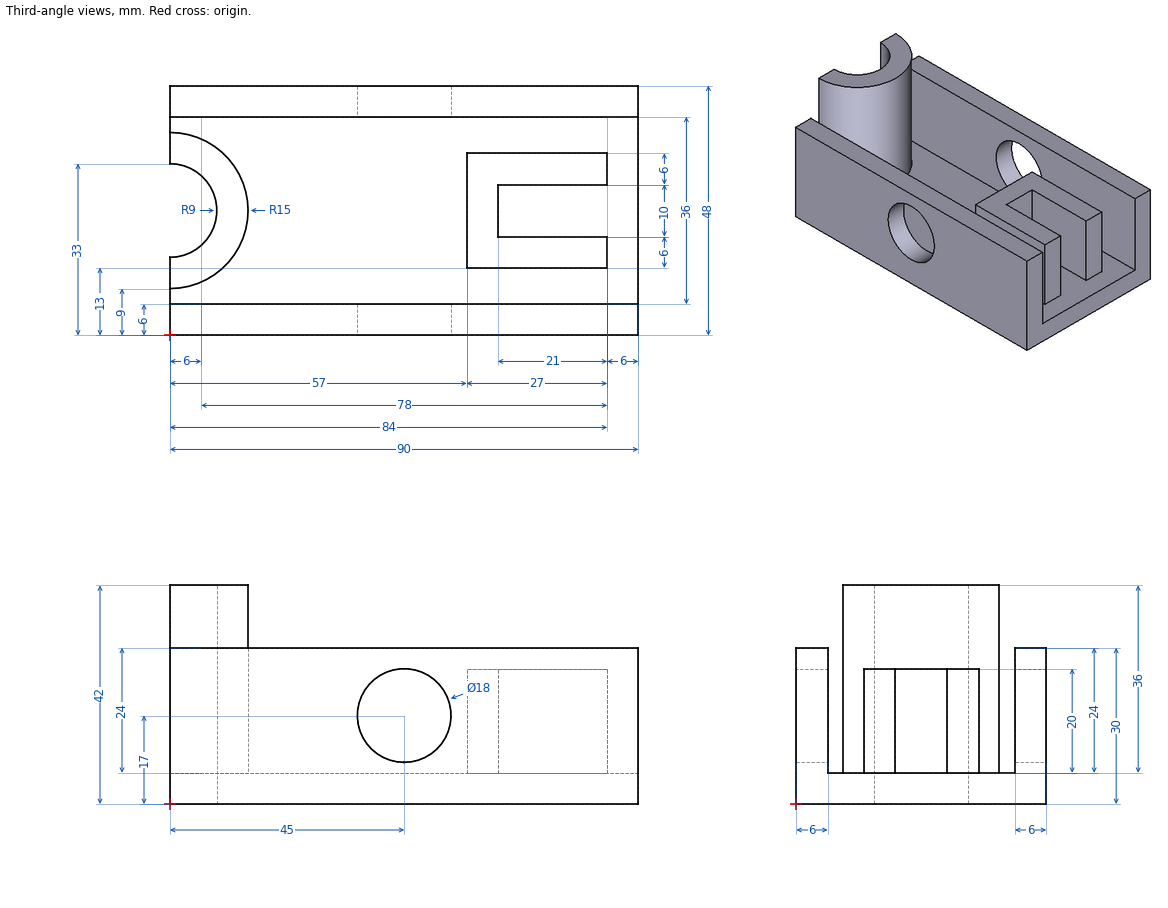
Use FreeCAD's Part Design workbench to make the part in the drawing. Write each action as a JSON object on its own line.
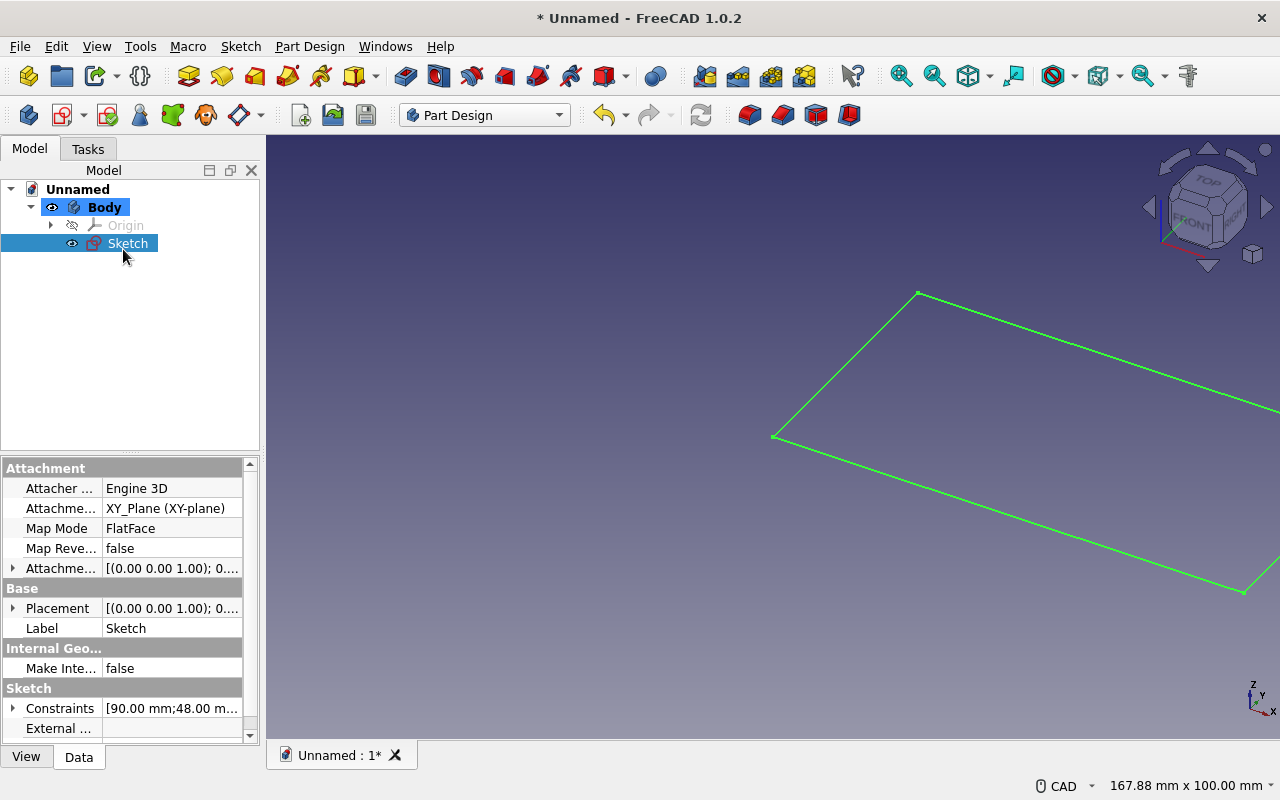
{"action": "left_click", "coordinate": [189, 76]}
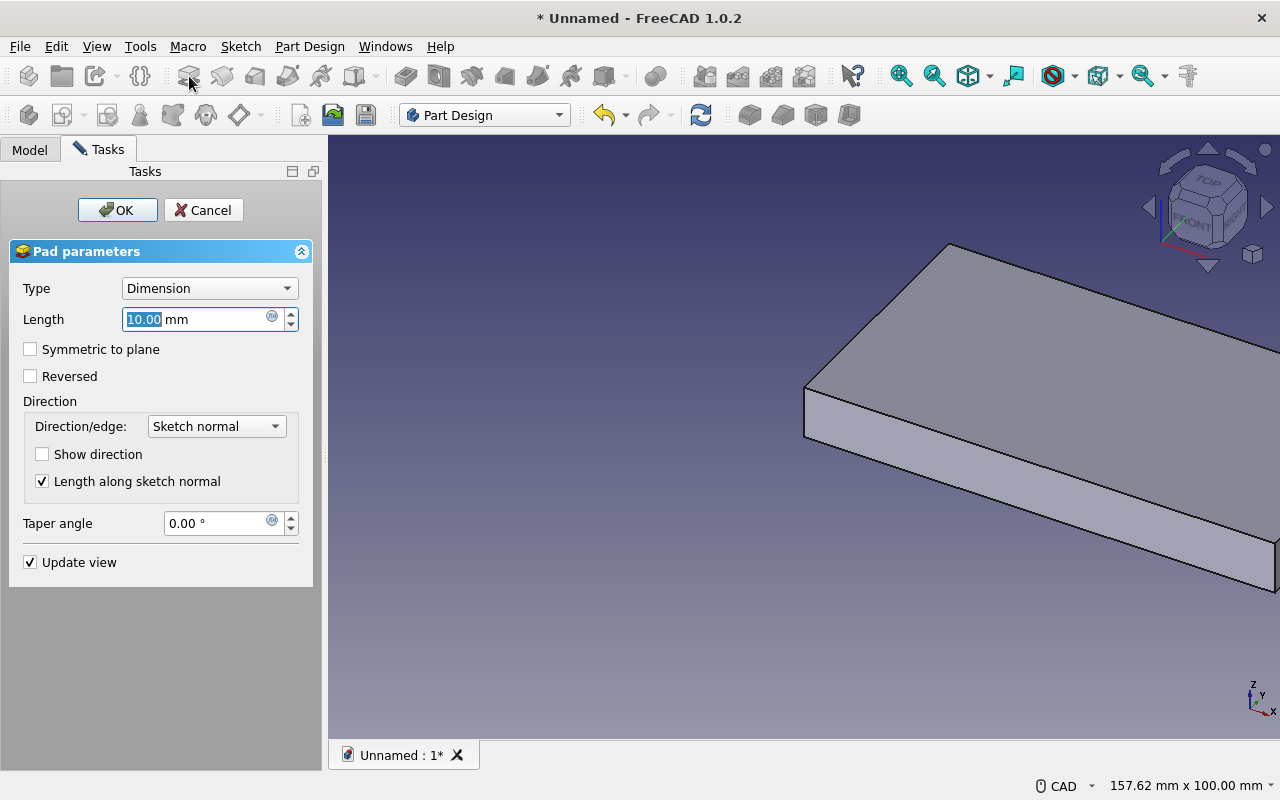
{"action": "type", "text": "30"}
{"action": "key", "text": "Tab"}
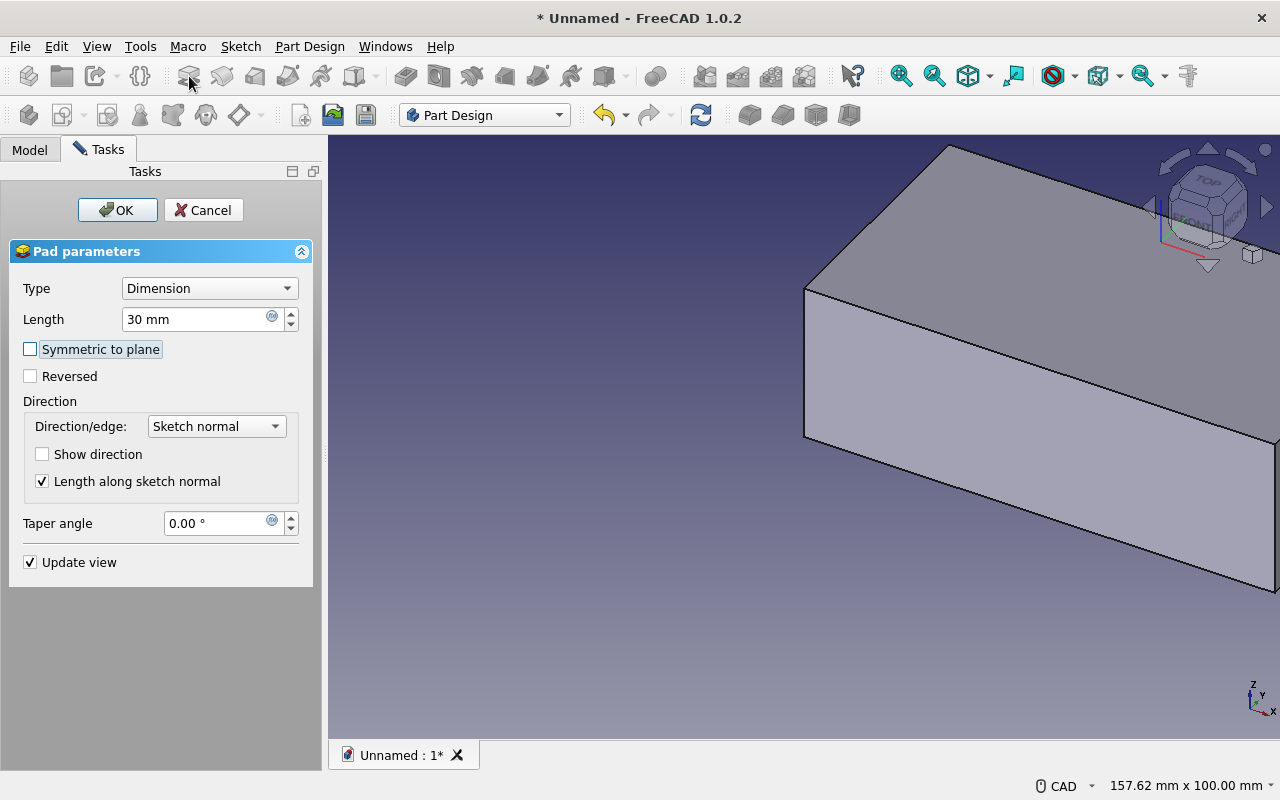
{"action": "left_click", "coordinate": [118, 210]}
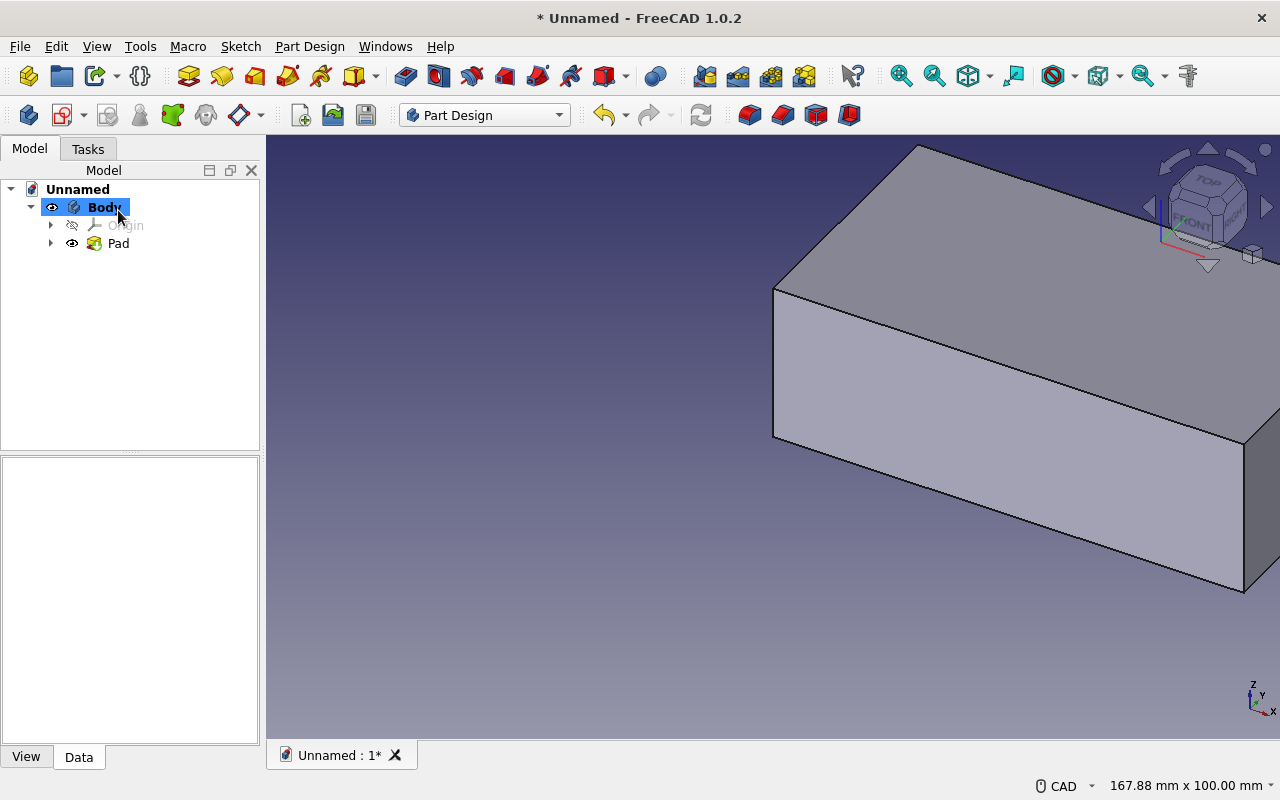
{"action": "left_click", "coordinate": [902, 76]}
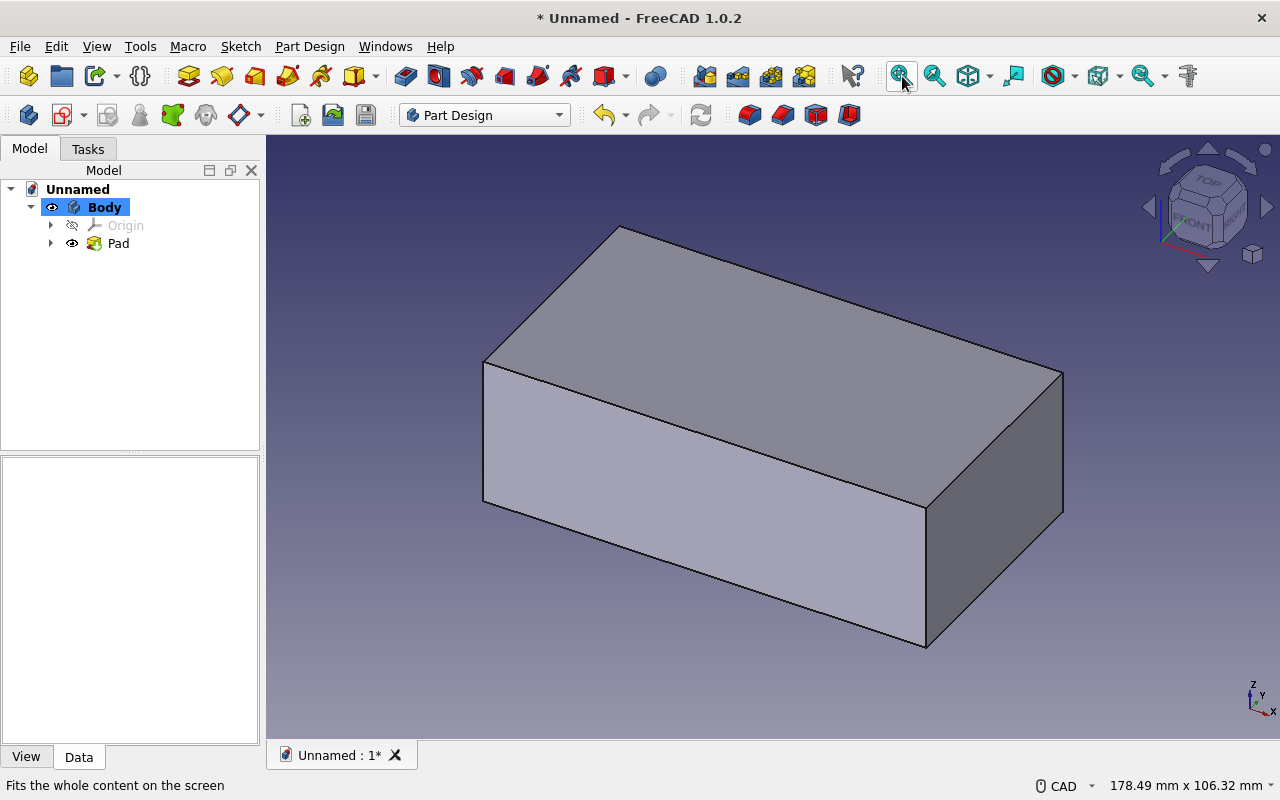
{"action": "left_click", "coordinate": [836, 387]}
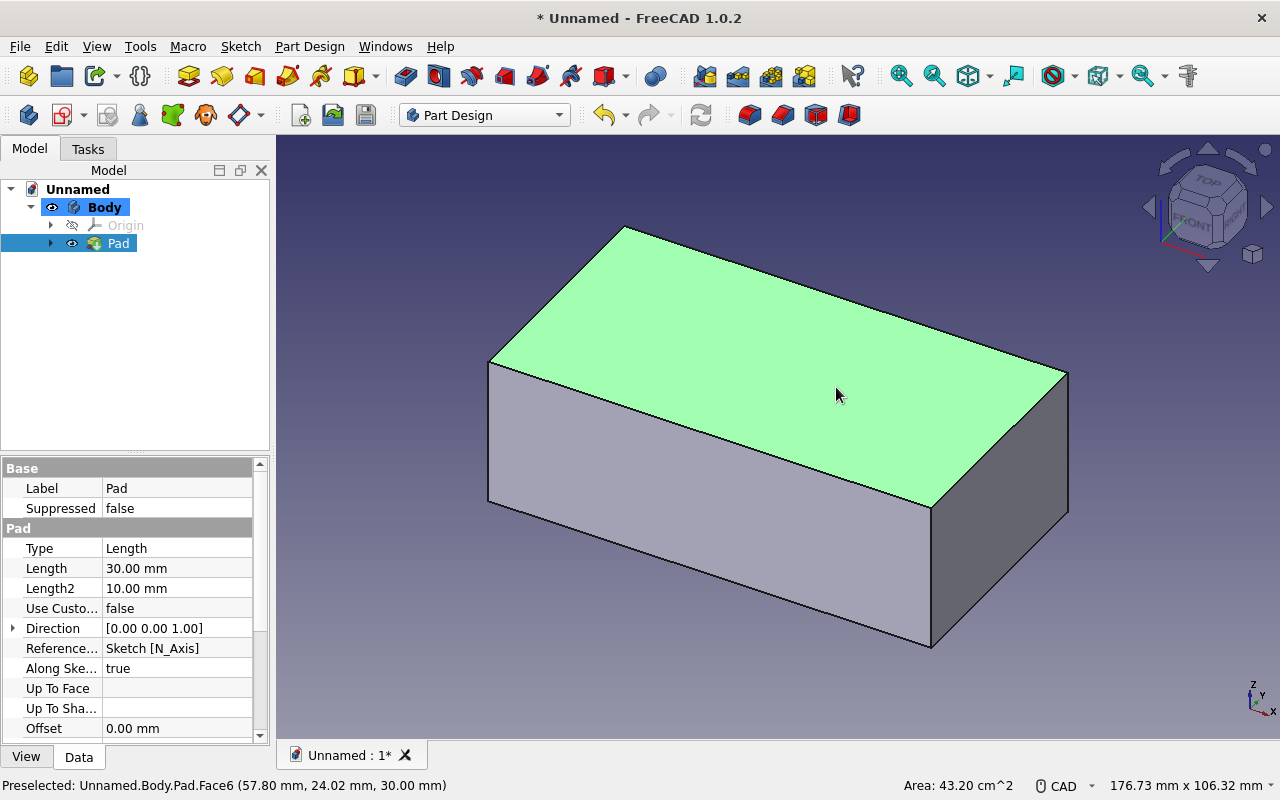
{"action": "left_click", "coordinate": [62, 116]}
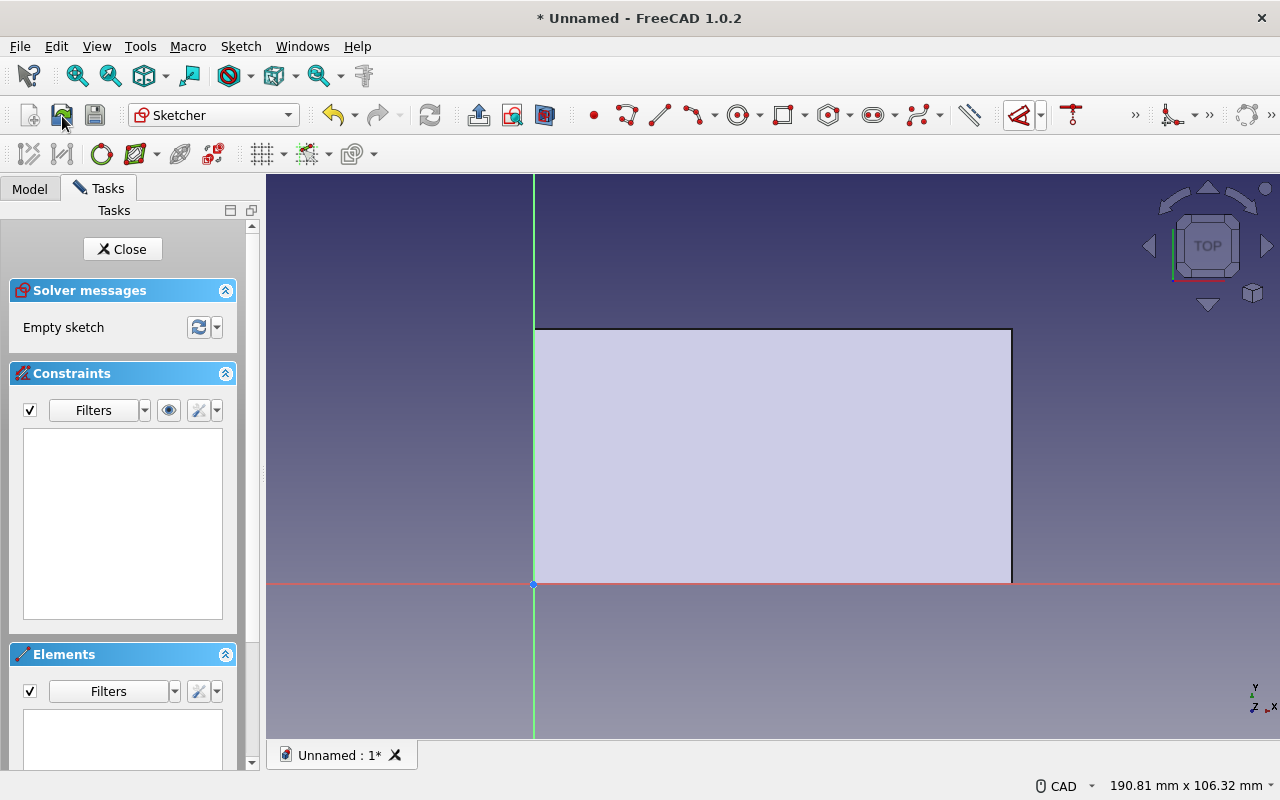
{"action": "key", "text": "g r"}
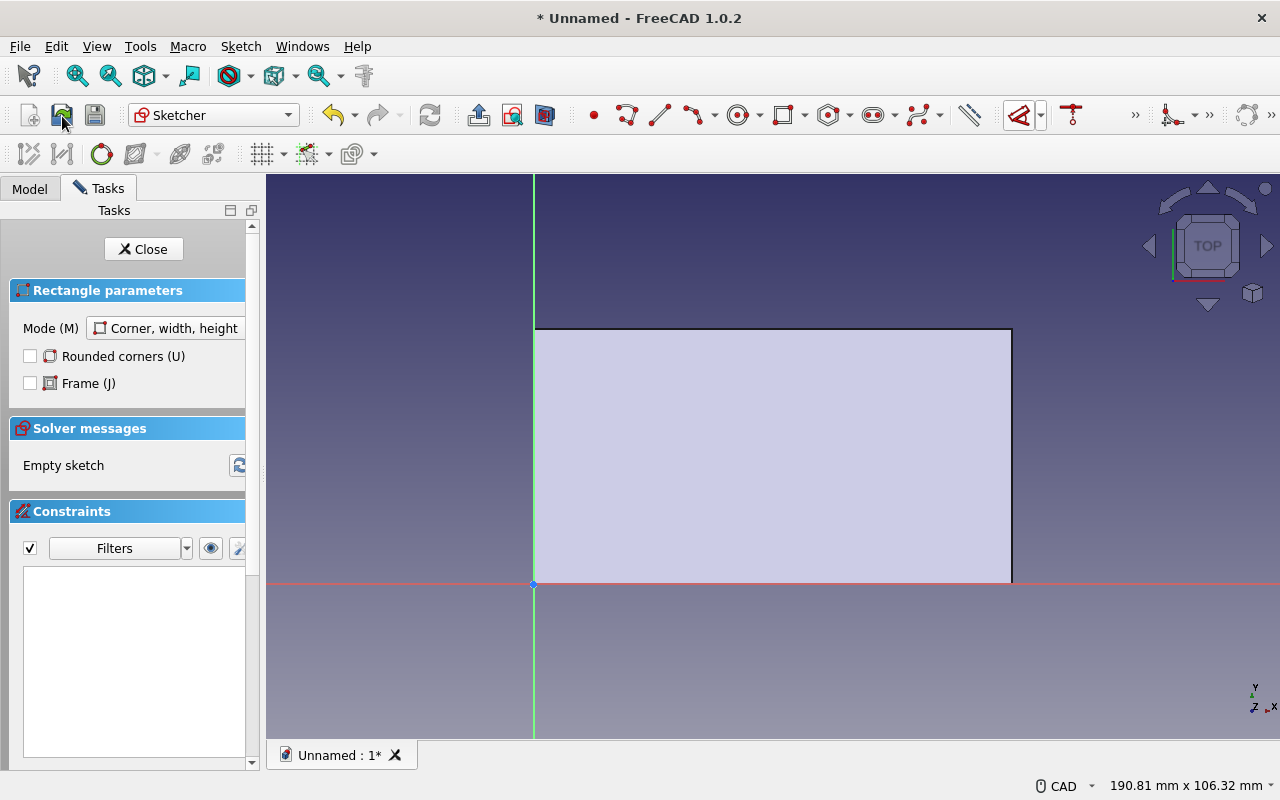
{"action": "left_click", "coordinate": [566, 361]}
{"action": "mouse_move", "coordinate": [980, 552]}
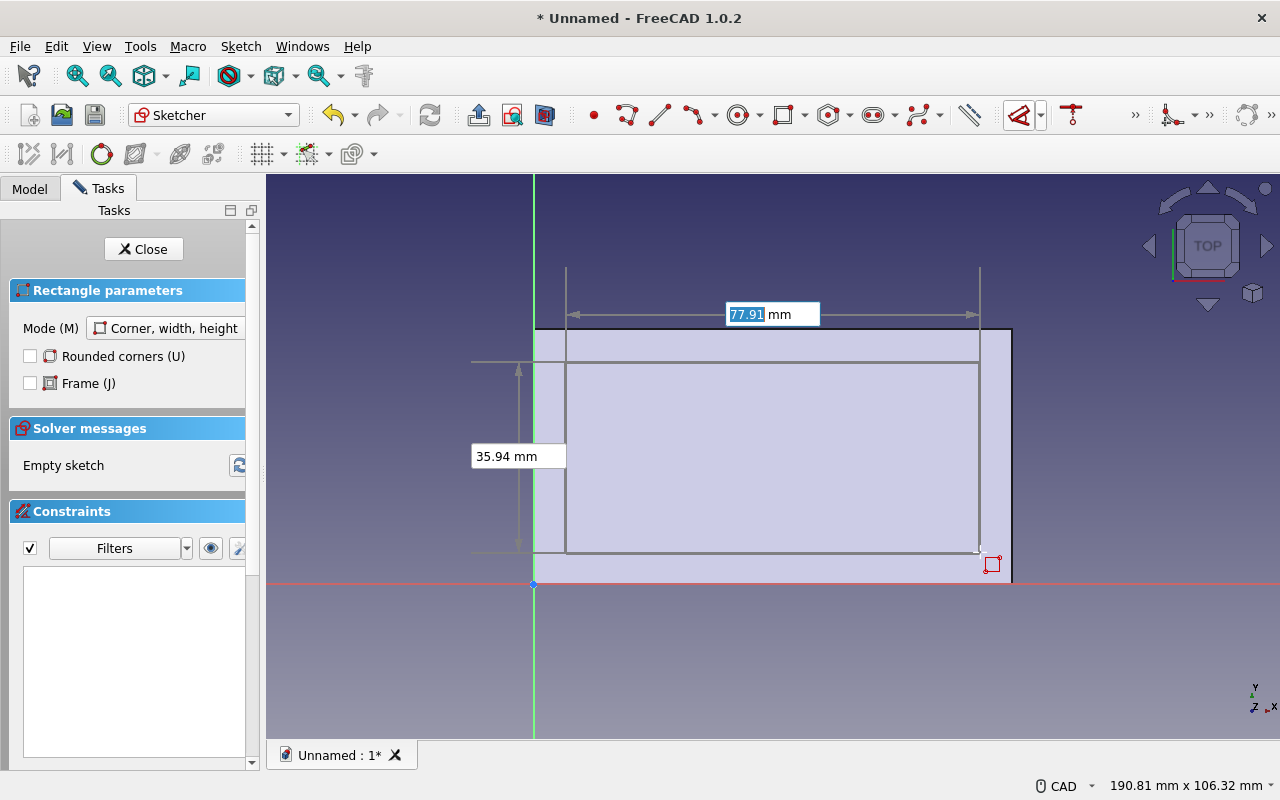
{"action": "type", "text": "78"}
{"action": "key", "text": "Tab"}
{"action": "type", "text": "36"}
{"action": "key", "text": "Return"}
{"action": "key", "text": "Escape"}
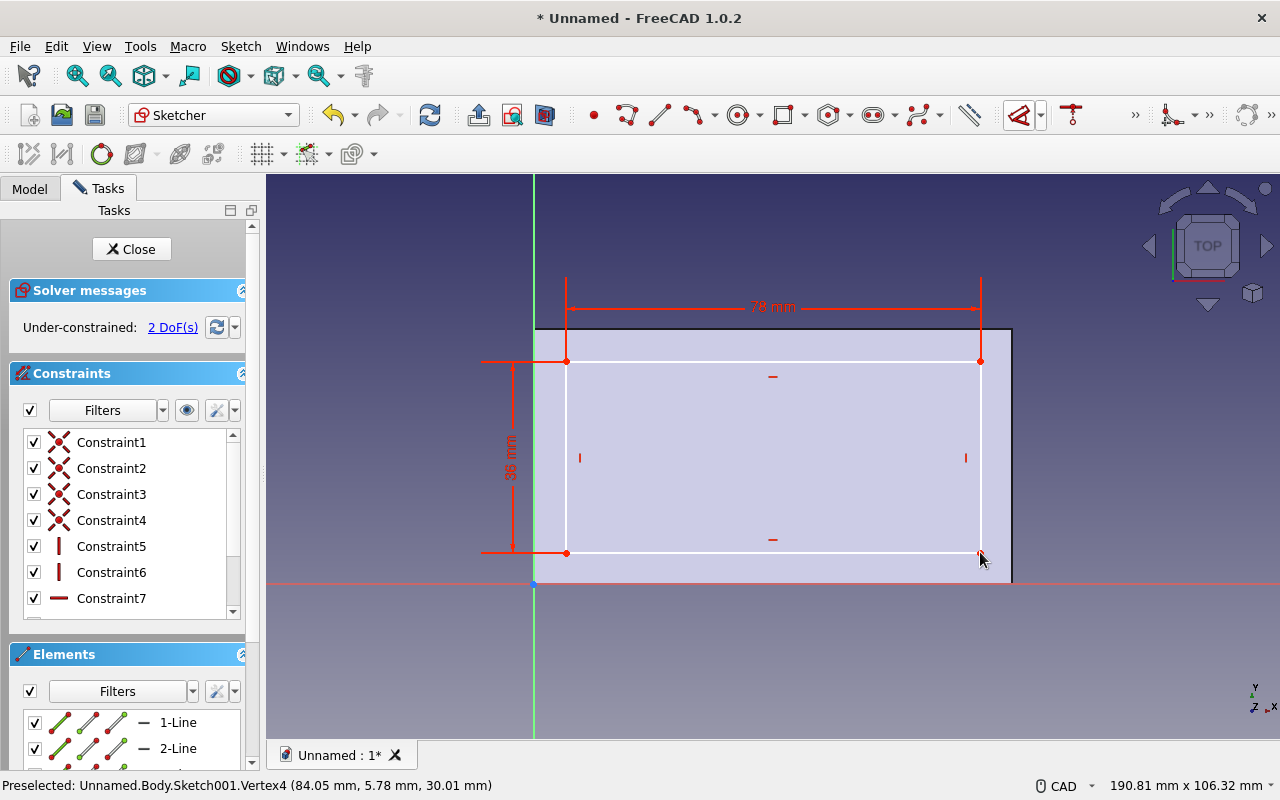
{"action": "key", "text": "d"}